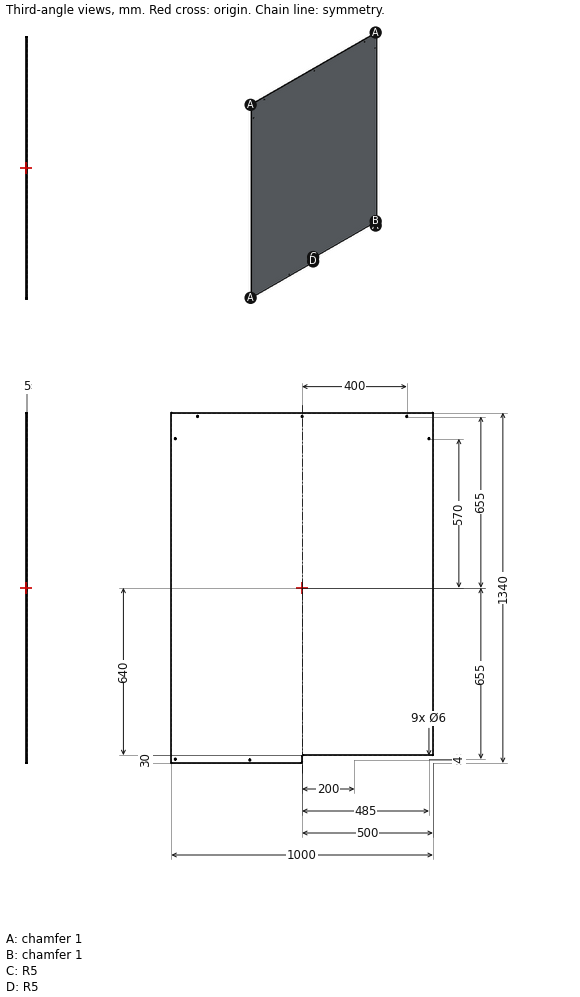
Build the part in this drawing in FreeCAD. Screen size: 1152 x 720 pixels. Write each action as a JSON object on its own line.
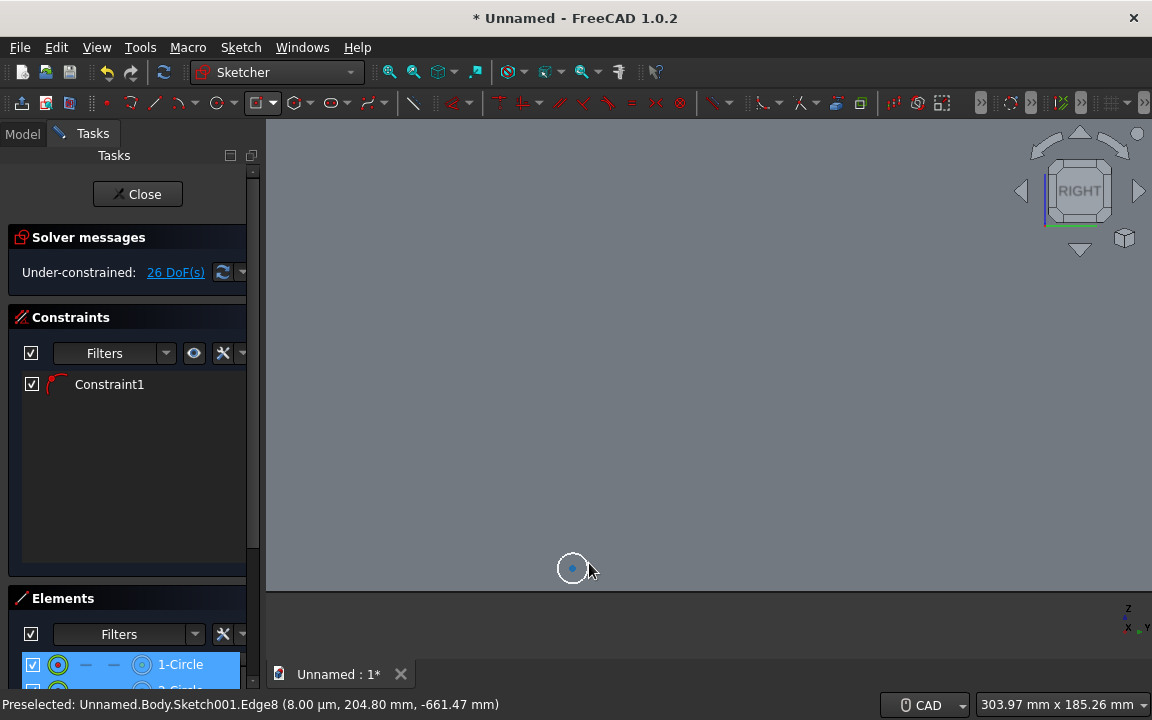
{"action": "left_click", "coordinate": [583, 558]}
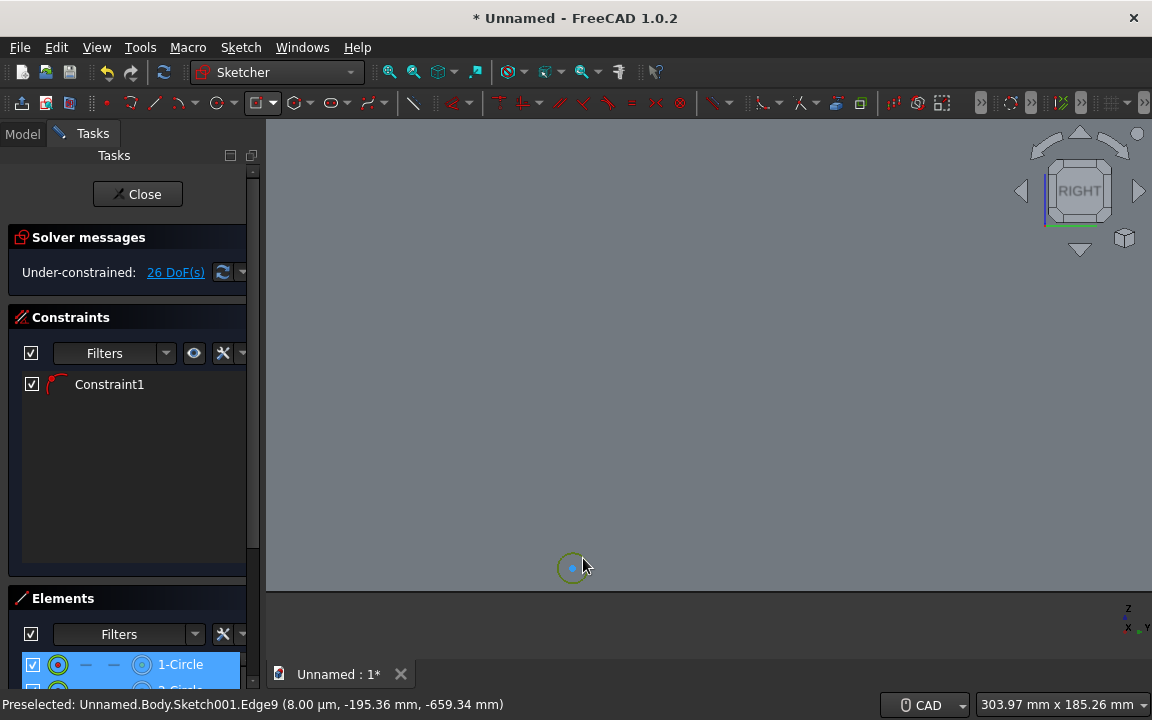
{"action": "left_click", "coordinate": [632, 104]}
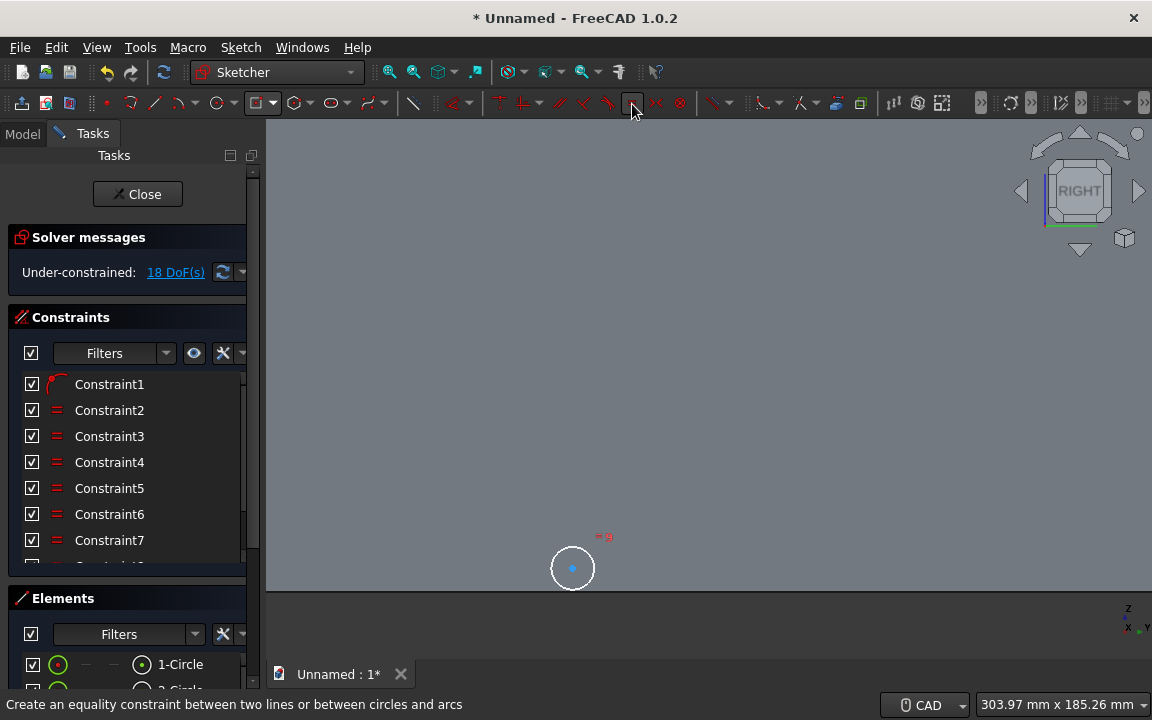
{"action": "scroll", "coordinate": [589, 563], "scroll_direction": "down", "scroll_amount": 12}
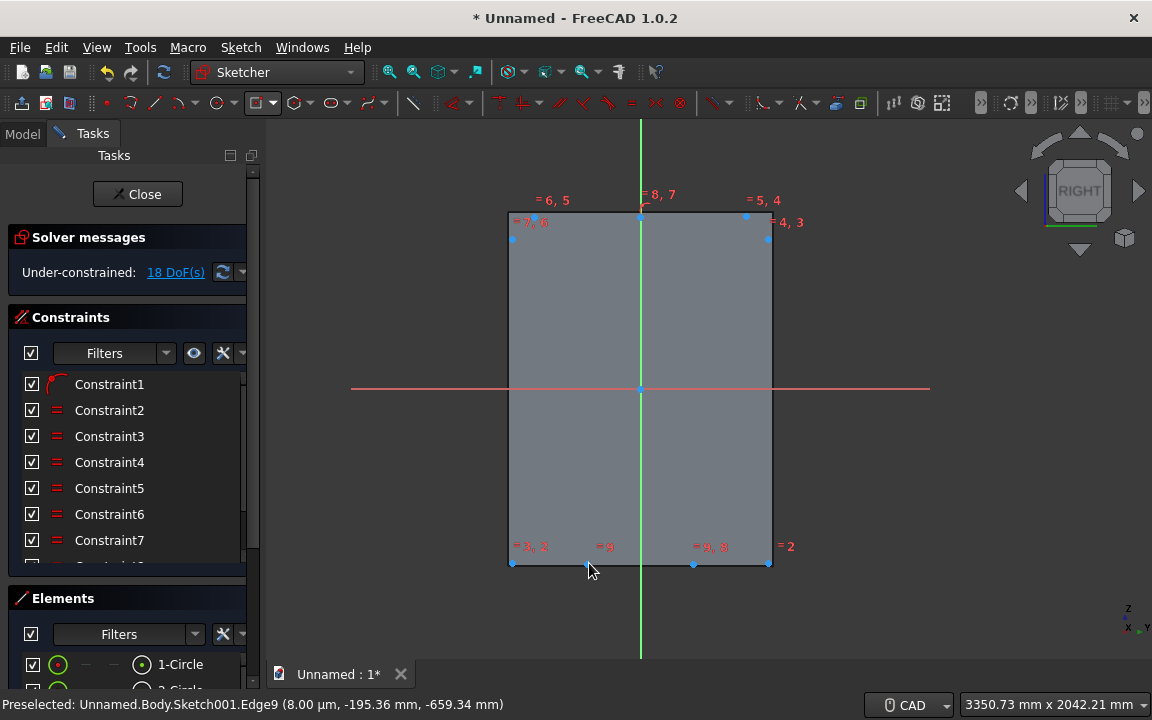
{"action": "left_click", "coordinate": [769, 564]}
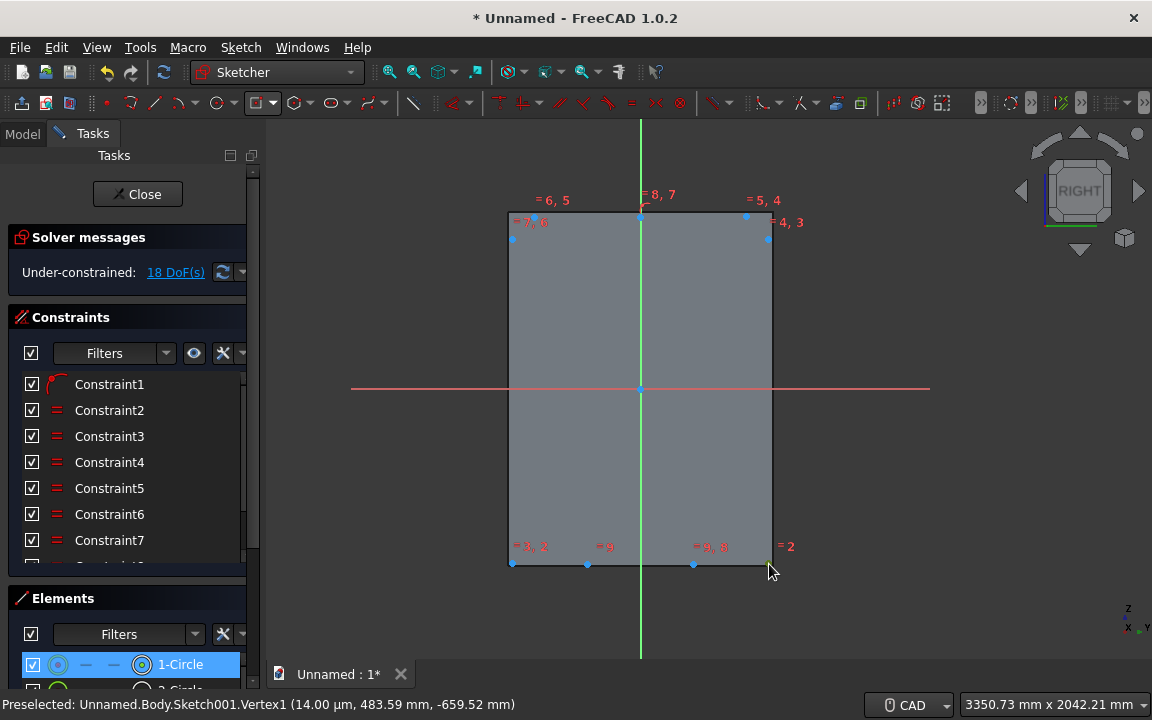
{"action": "left_click", "coordinate": [513, 564]}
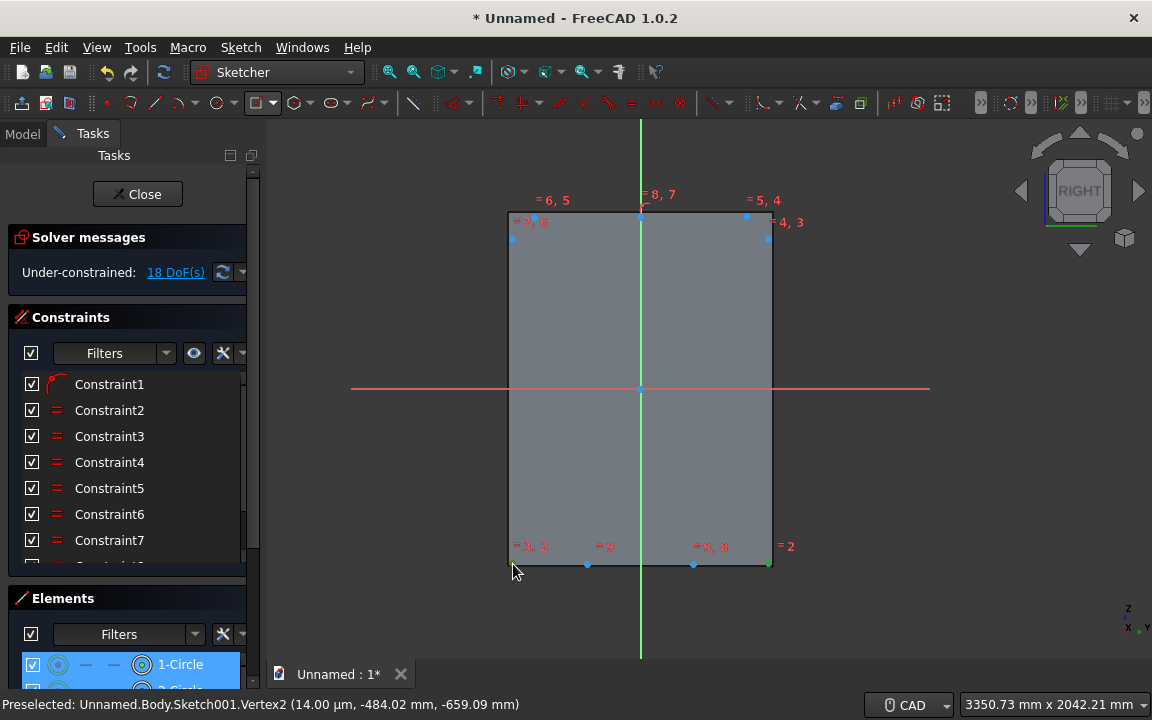
{"action": "left_click", "coordinate": [641, 596]}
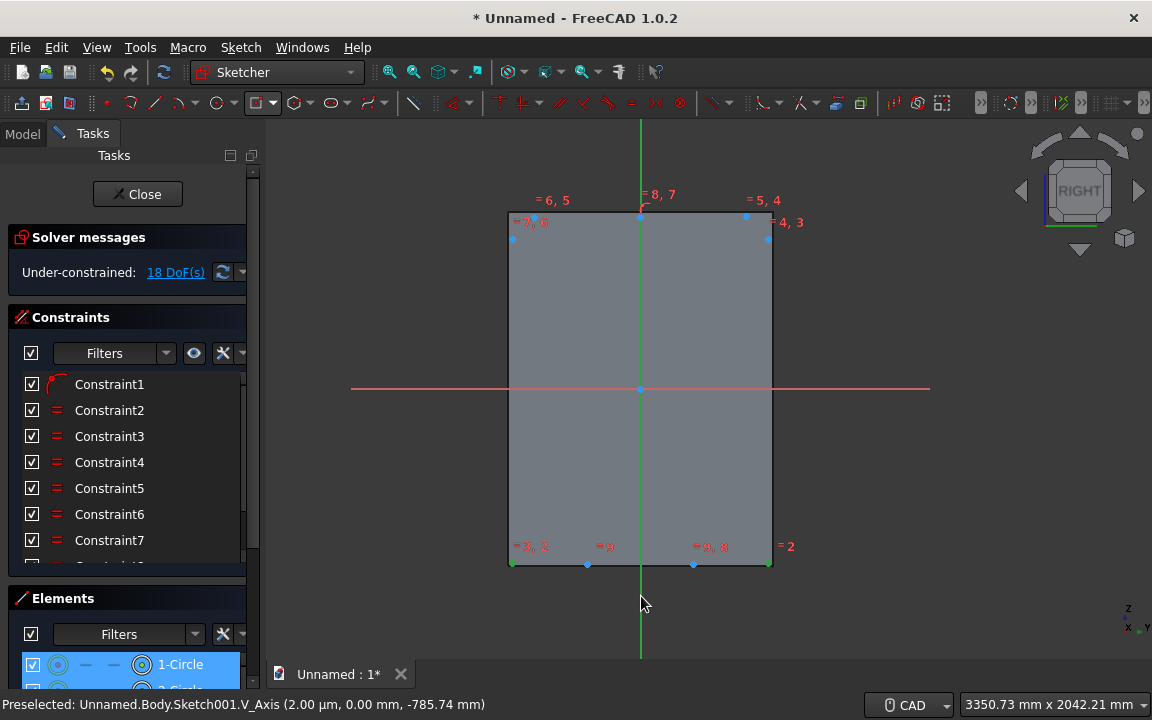
{"action": "left_click", "coordinate": [656, 104]}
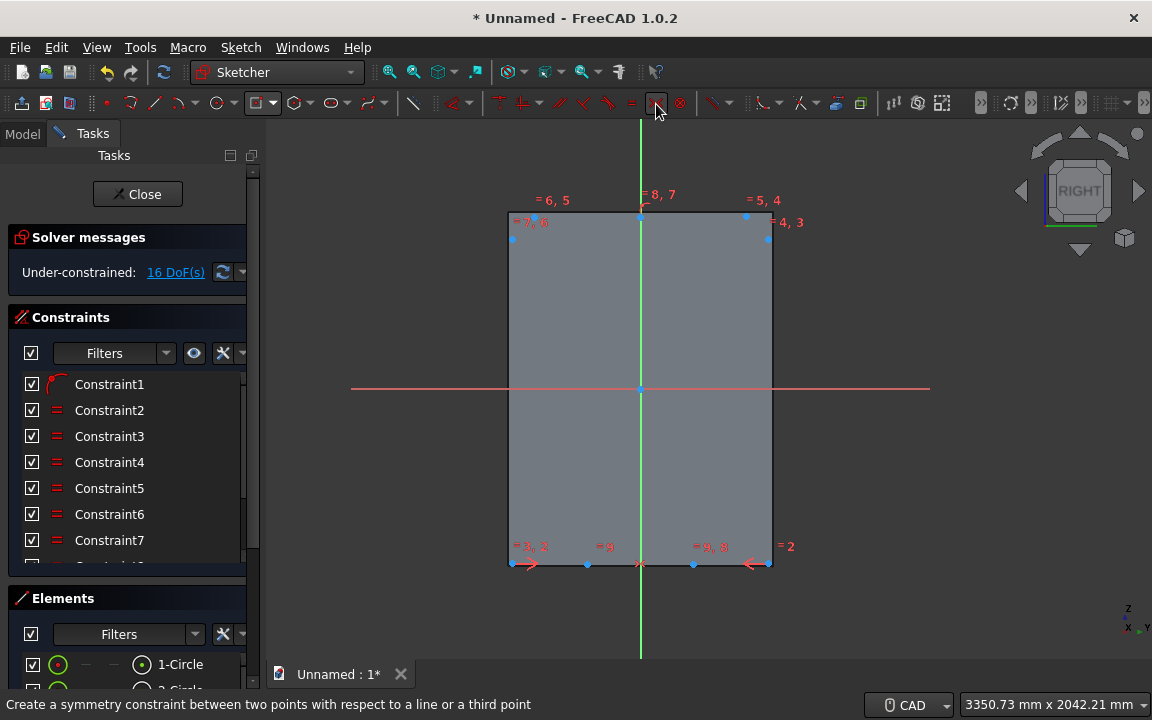
{"action": "left_click", "coordinate": [746, 217]}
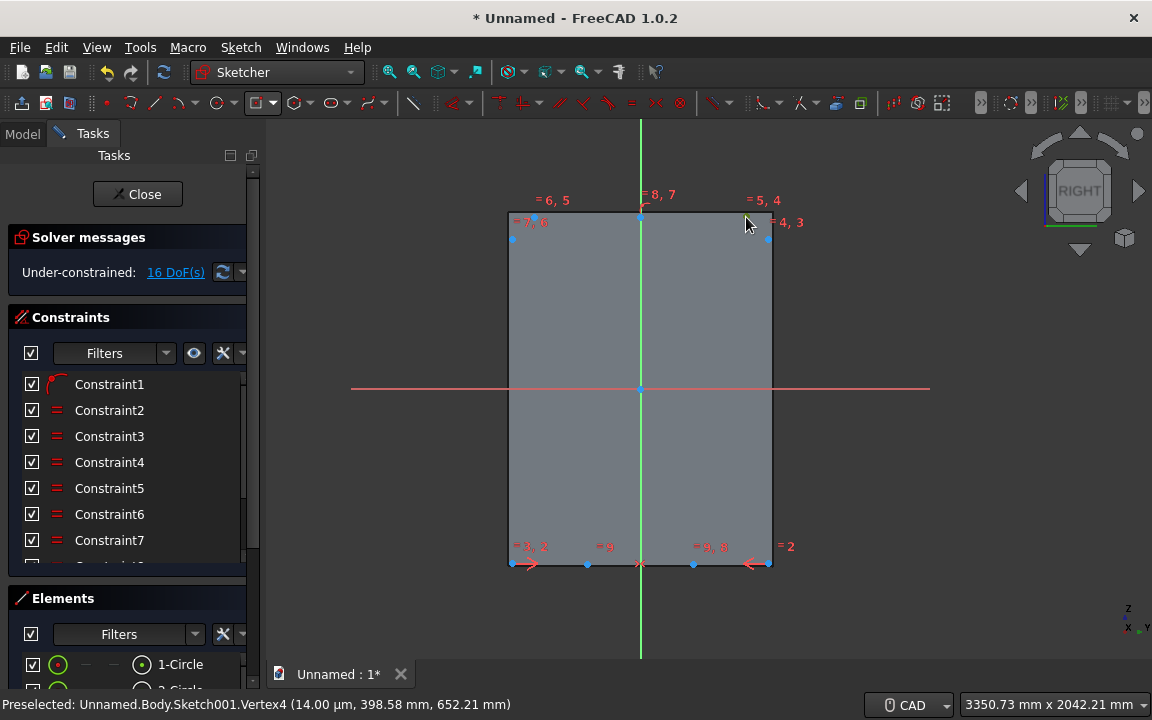
{"action": "left_click", "coordinate": [535, 217]}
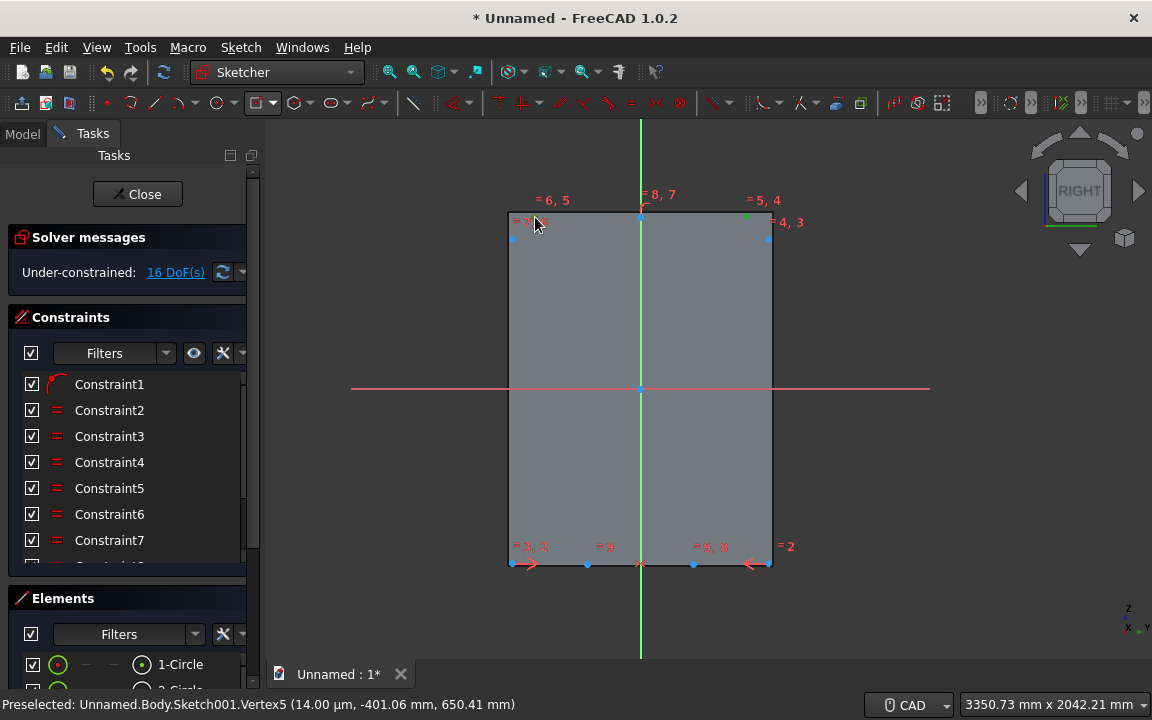
{"action": "left_click", "coordinate": [641, 596]}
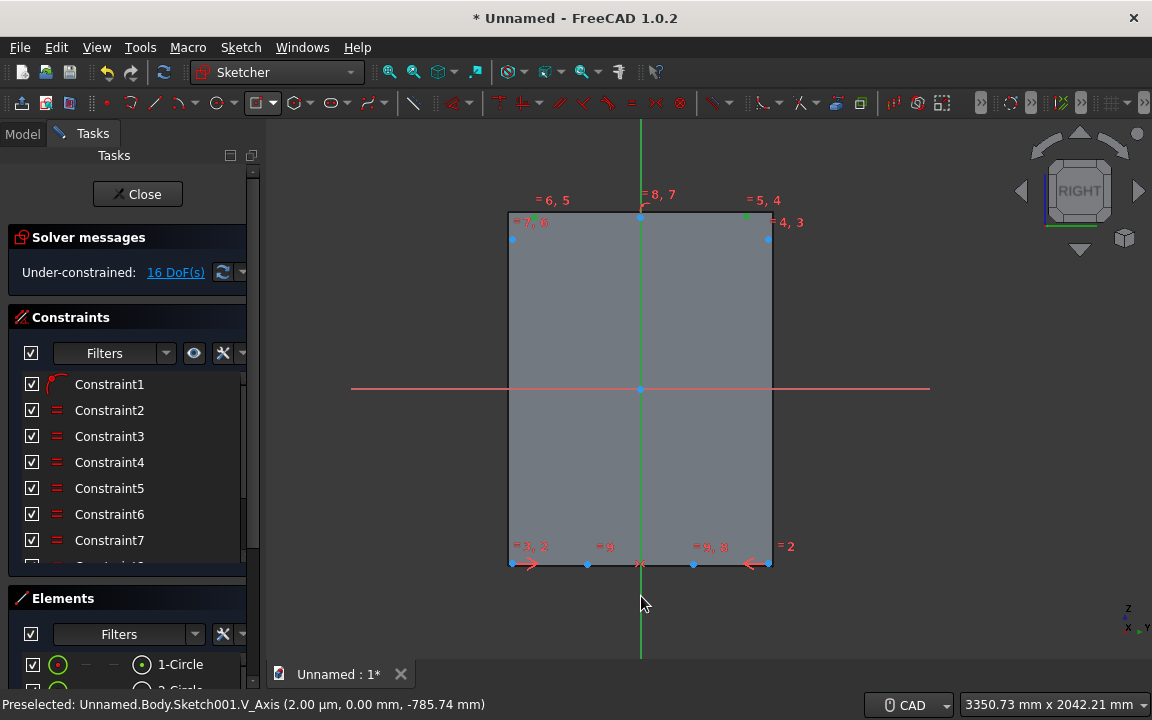
{"action": "left_click", "coordinate": [656, 104]}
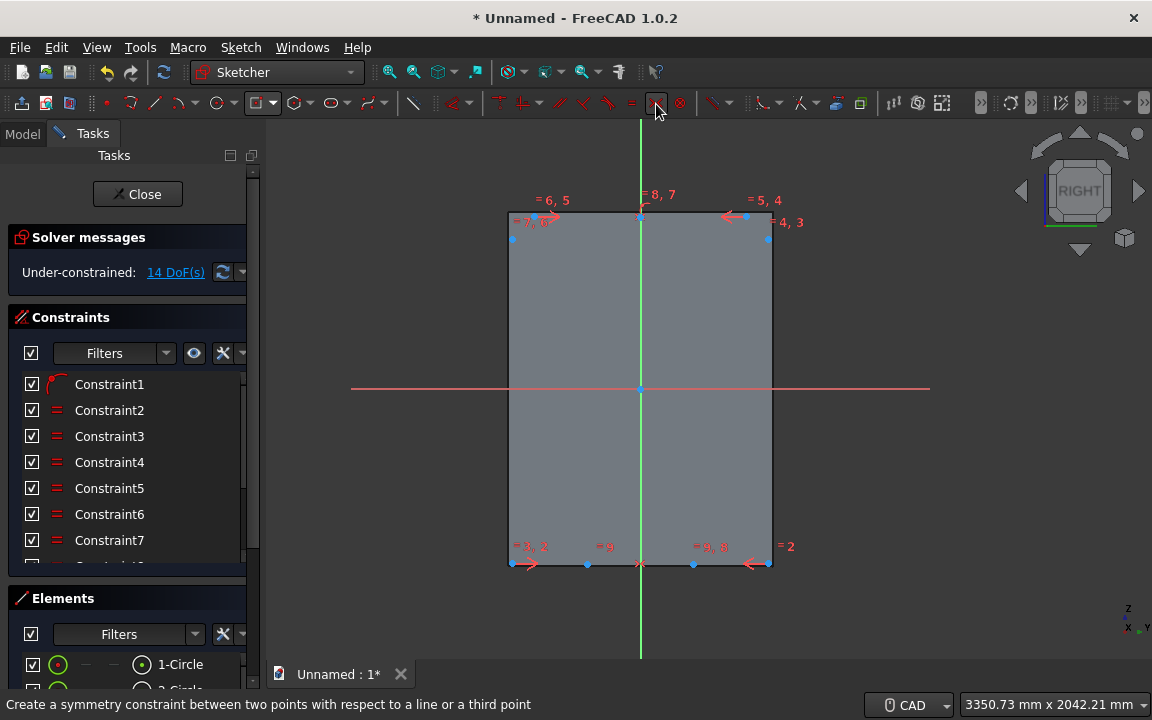
{"action": "left_click", "coordinate": [769, 239]}